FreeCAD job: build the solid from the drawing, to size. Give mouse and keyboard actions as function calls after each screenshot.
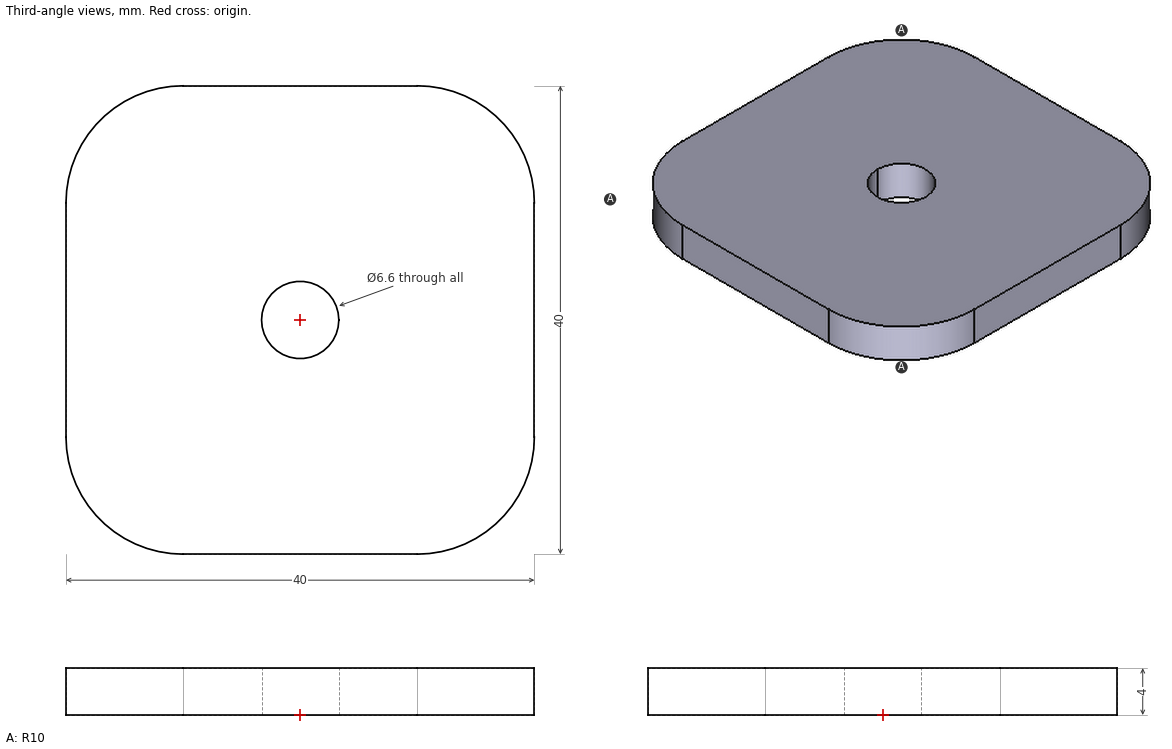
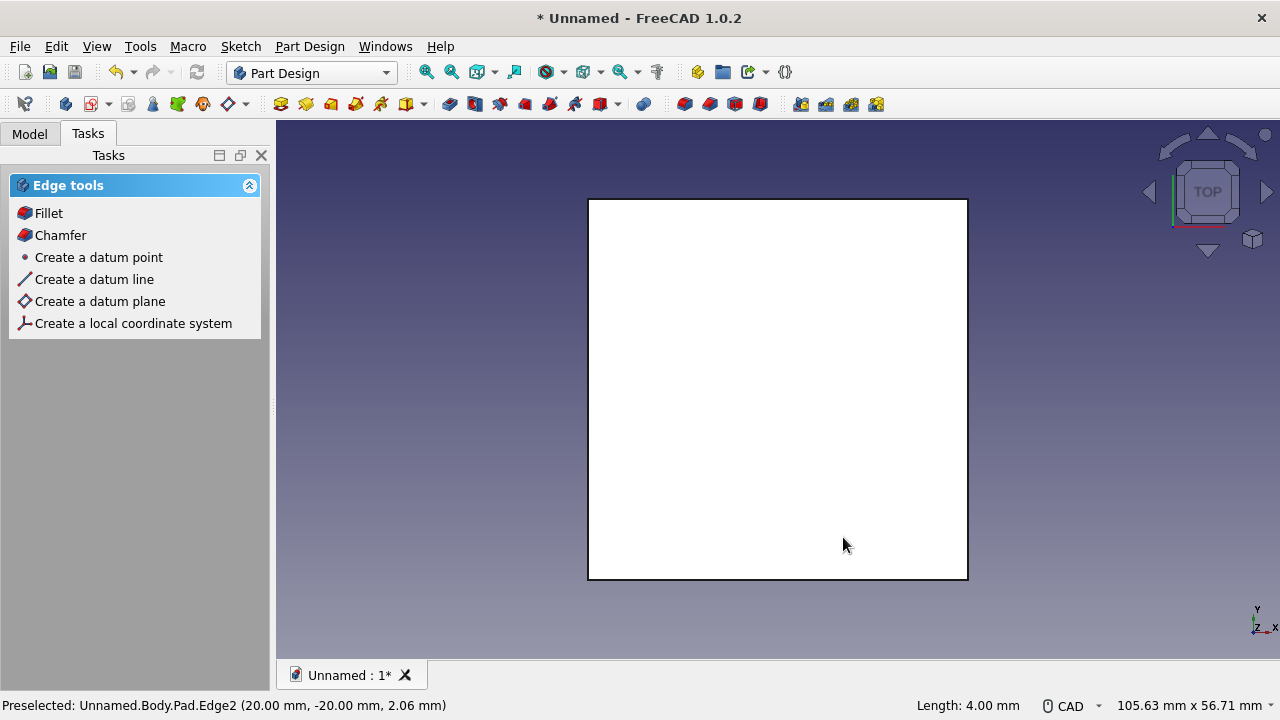
key(1)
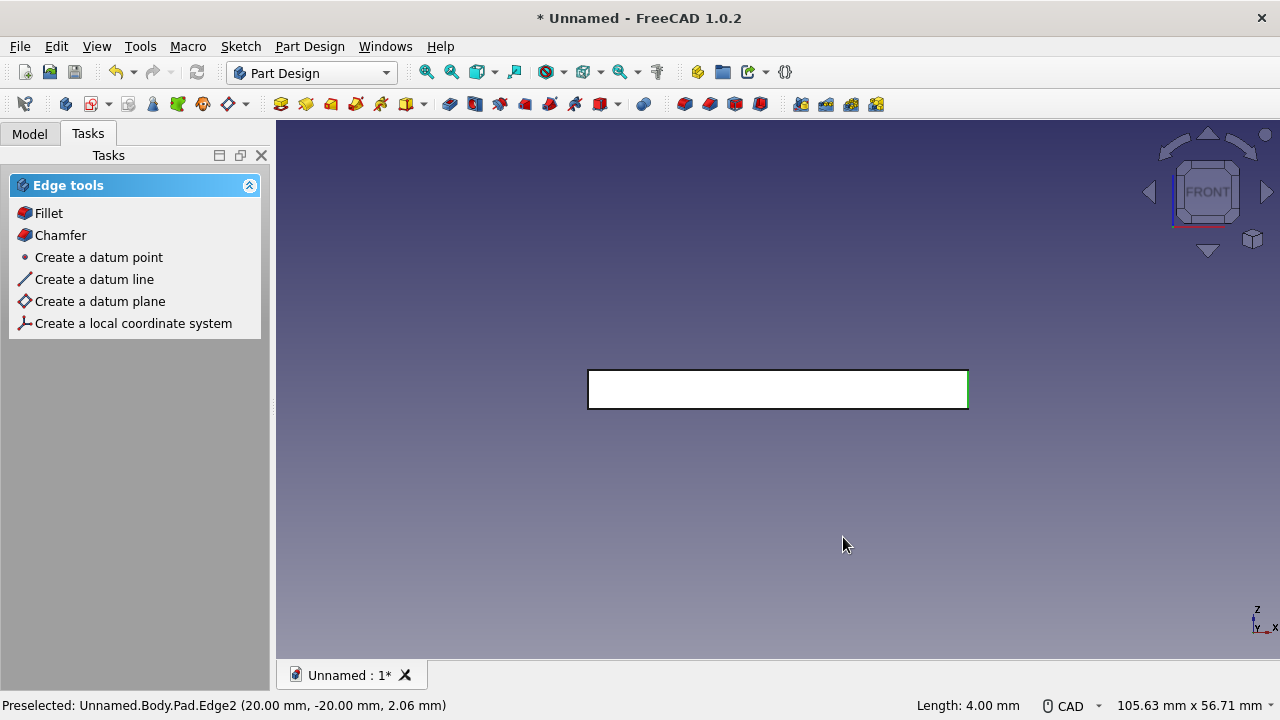
click(427, 72)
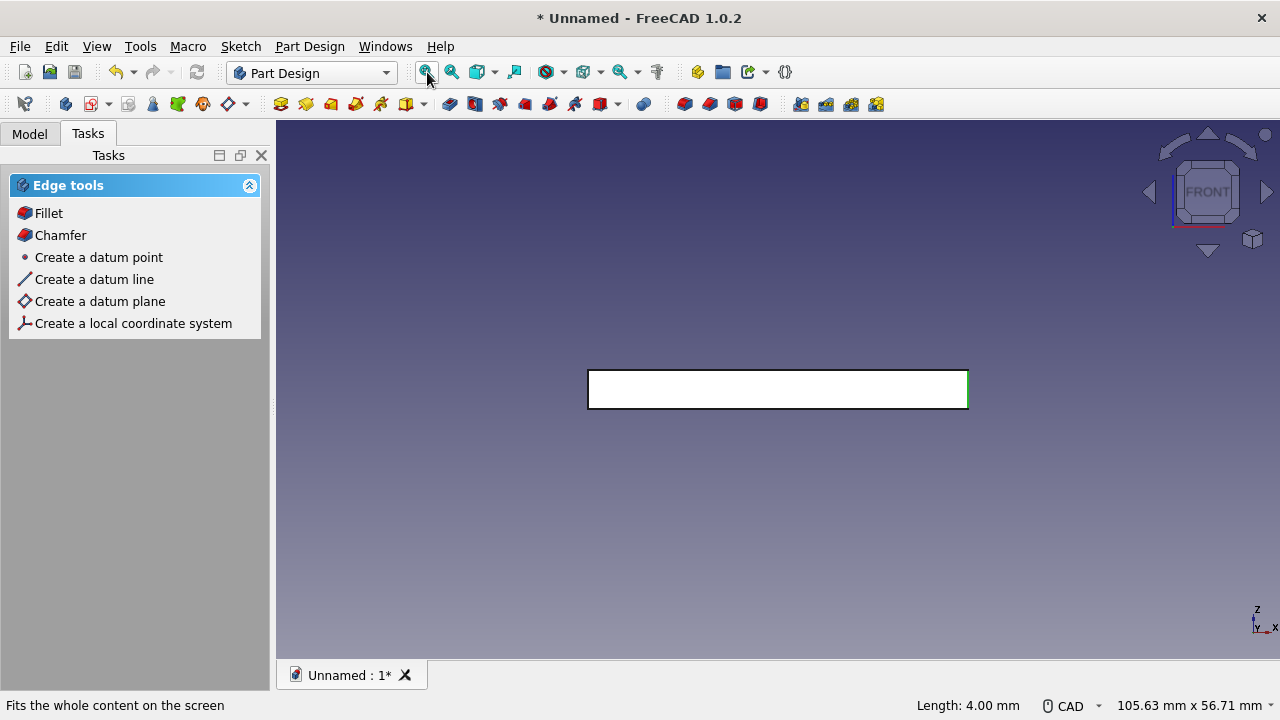
click(588, 389, ctrl)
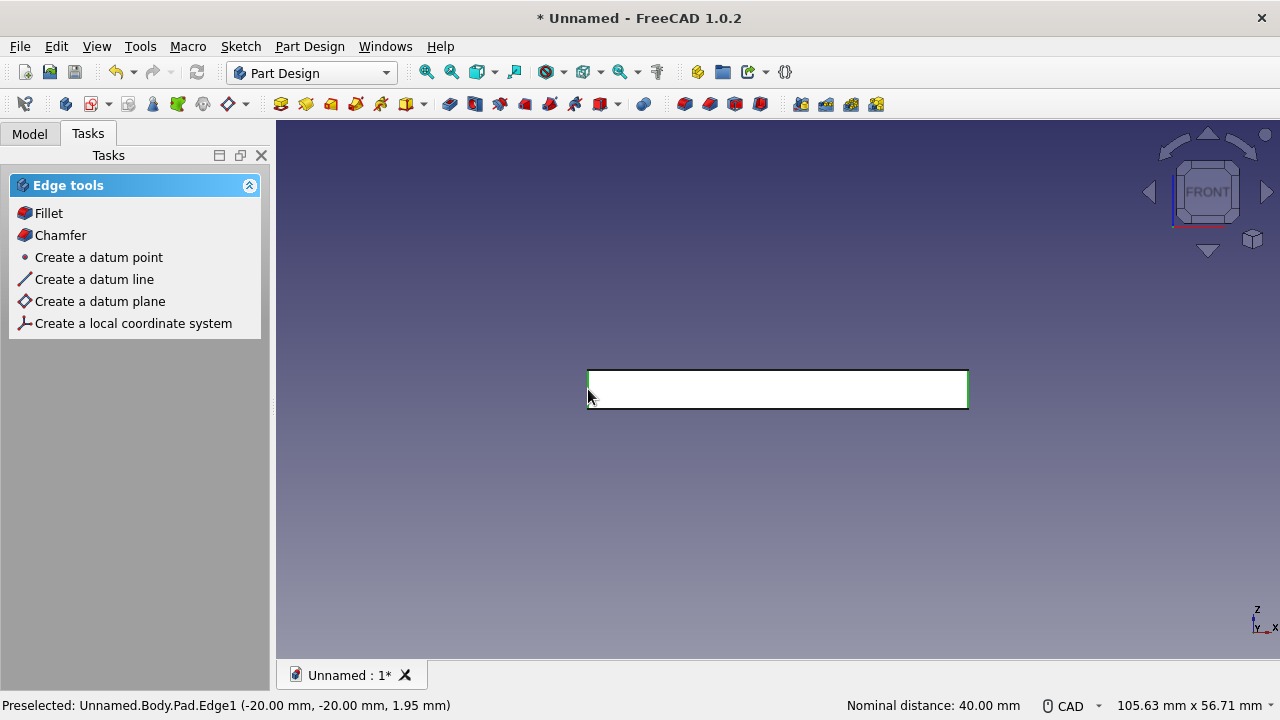
key(3)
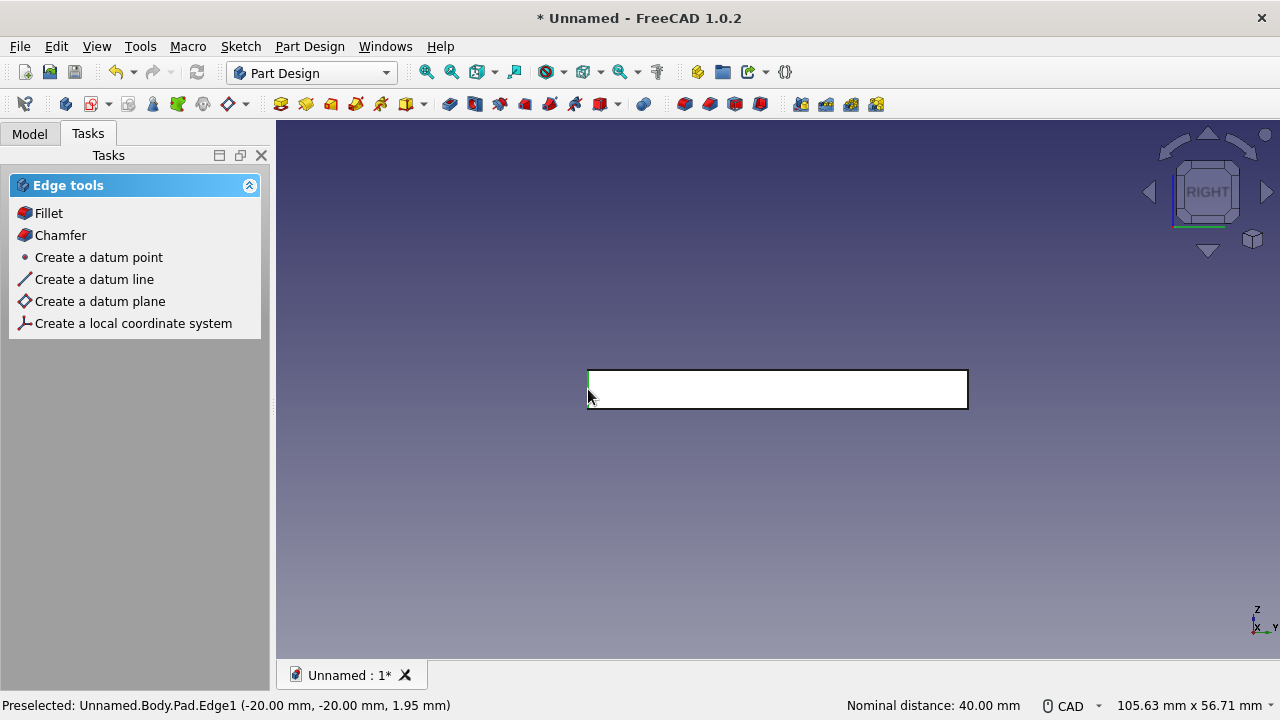
click(427, 72)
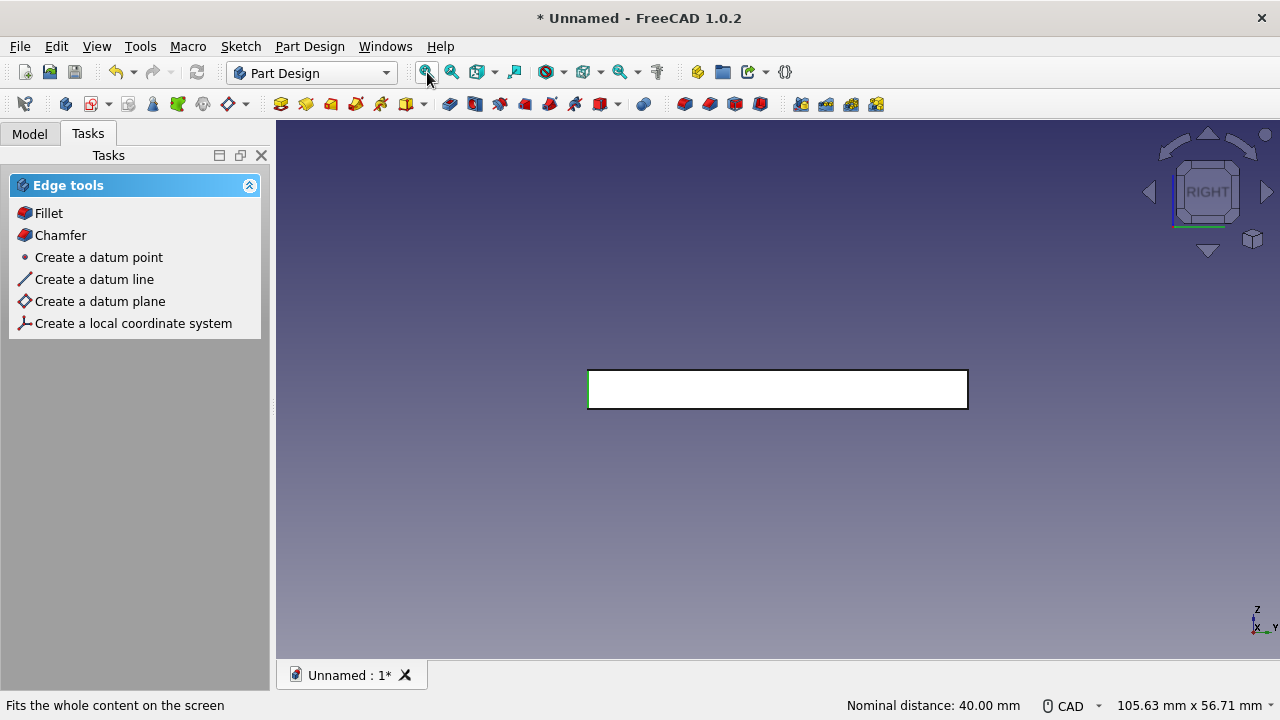
click(968, 388, ctrl)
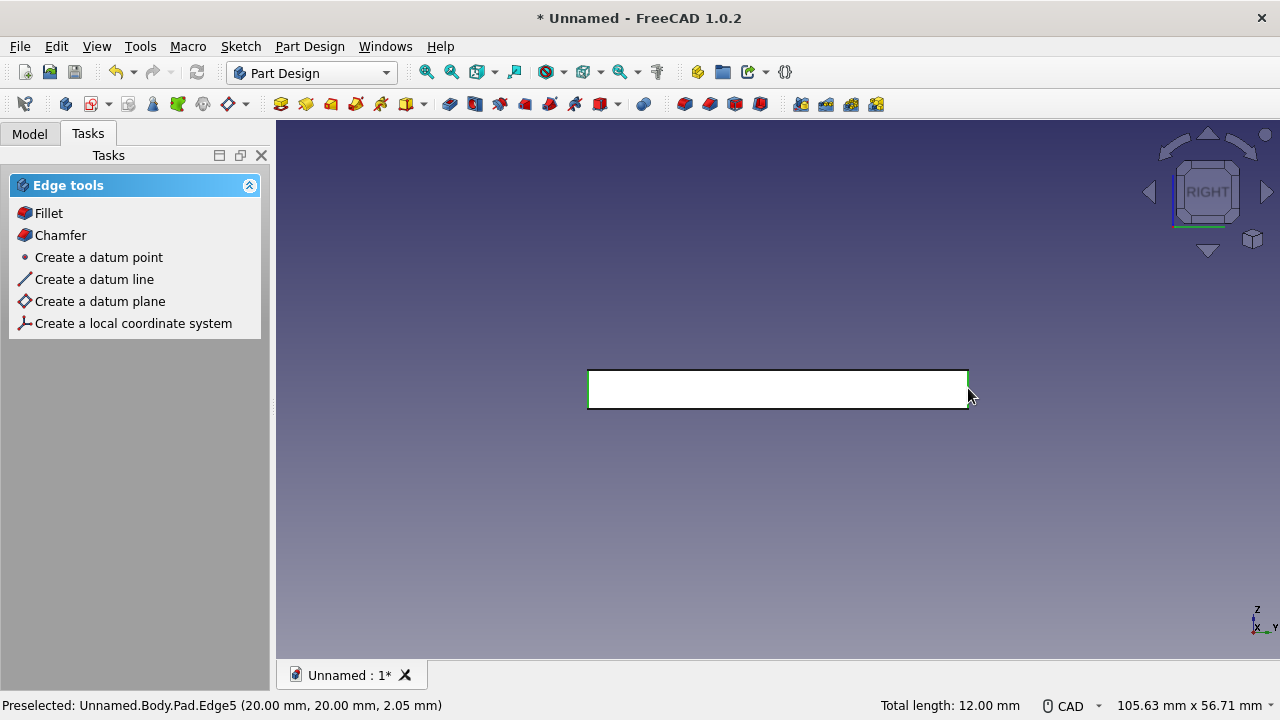
key(5)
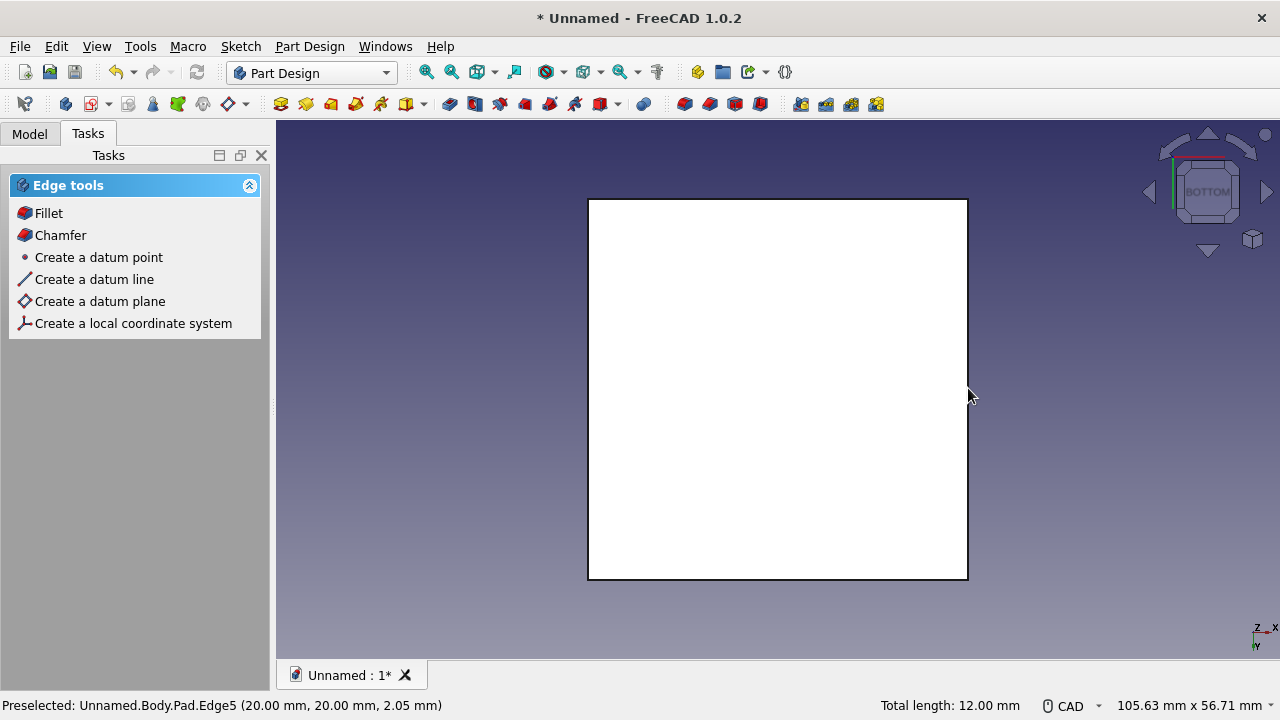
key(4)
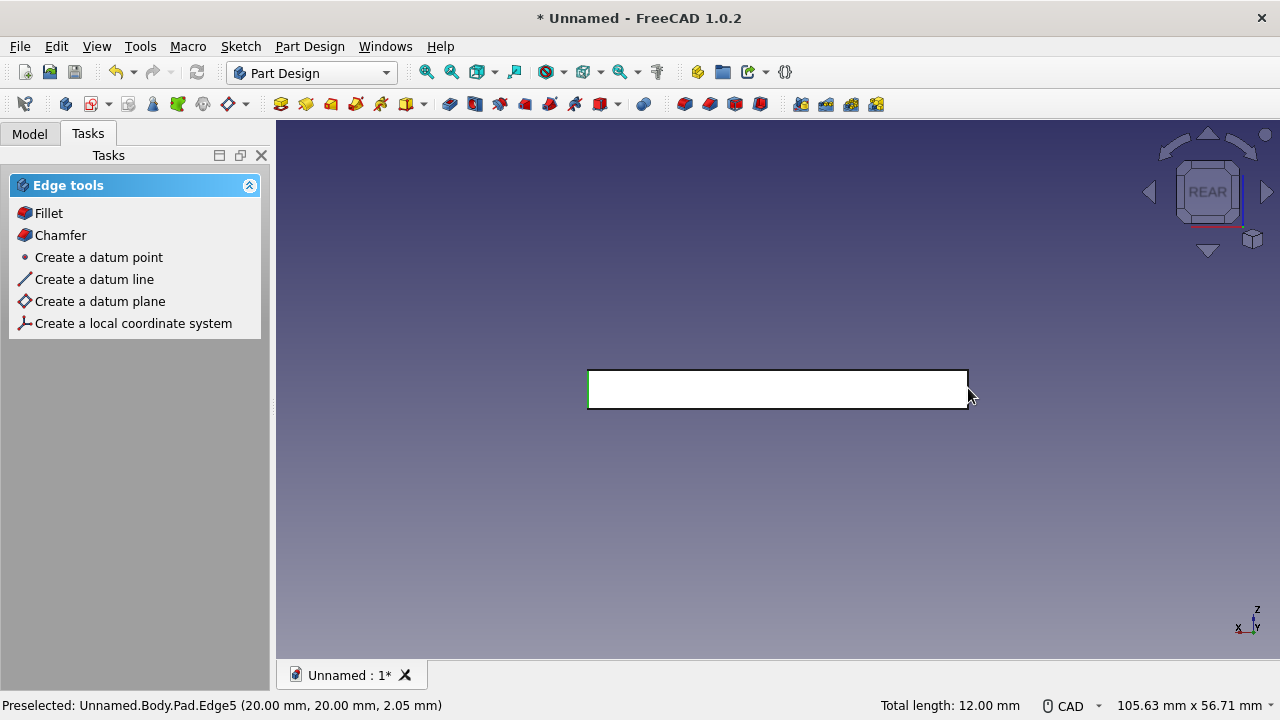
click(427, 72)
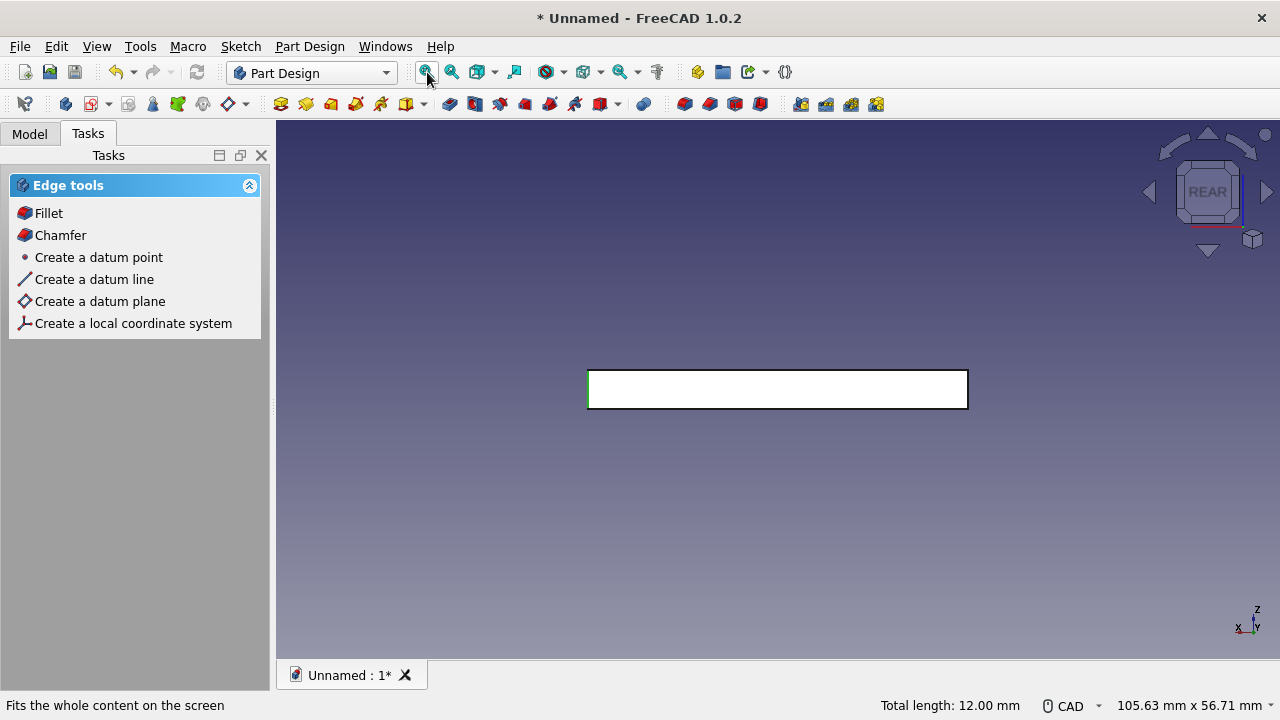
click(968, 389, ctrl)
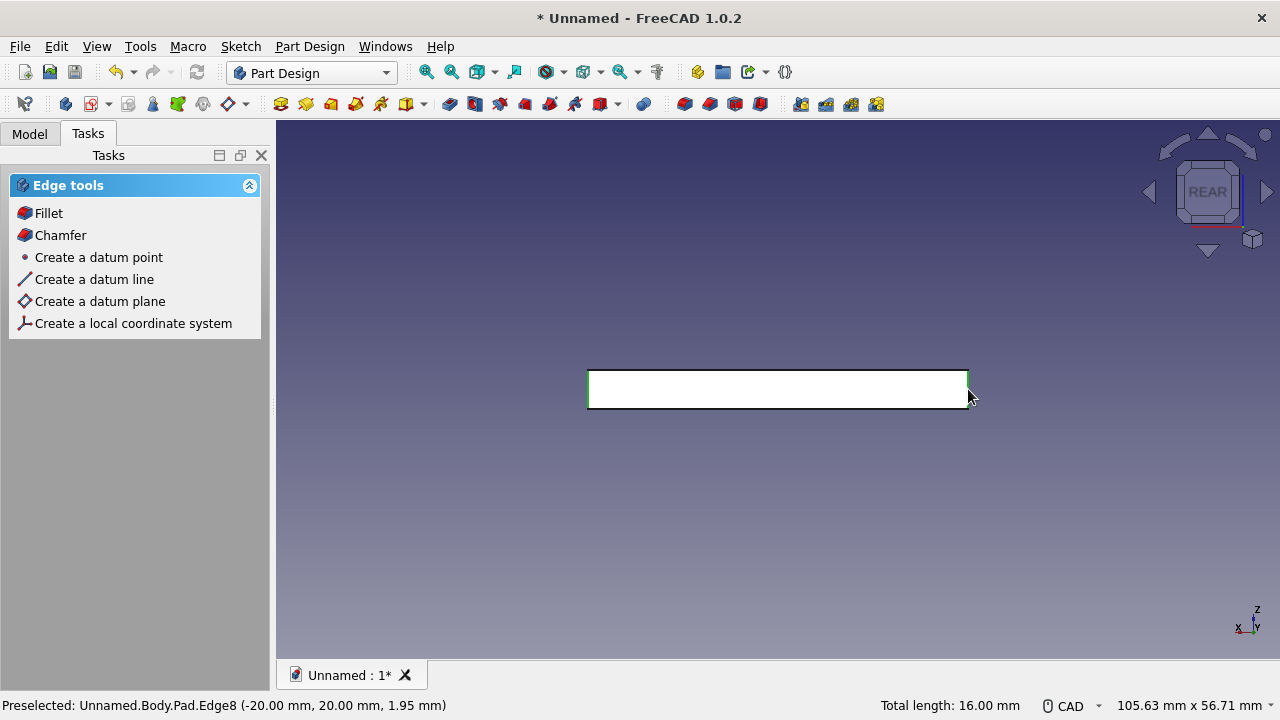
click(685, 104)